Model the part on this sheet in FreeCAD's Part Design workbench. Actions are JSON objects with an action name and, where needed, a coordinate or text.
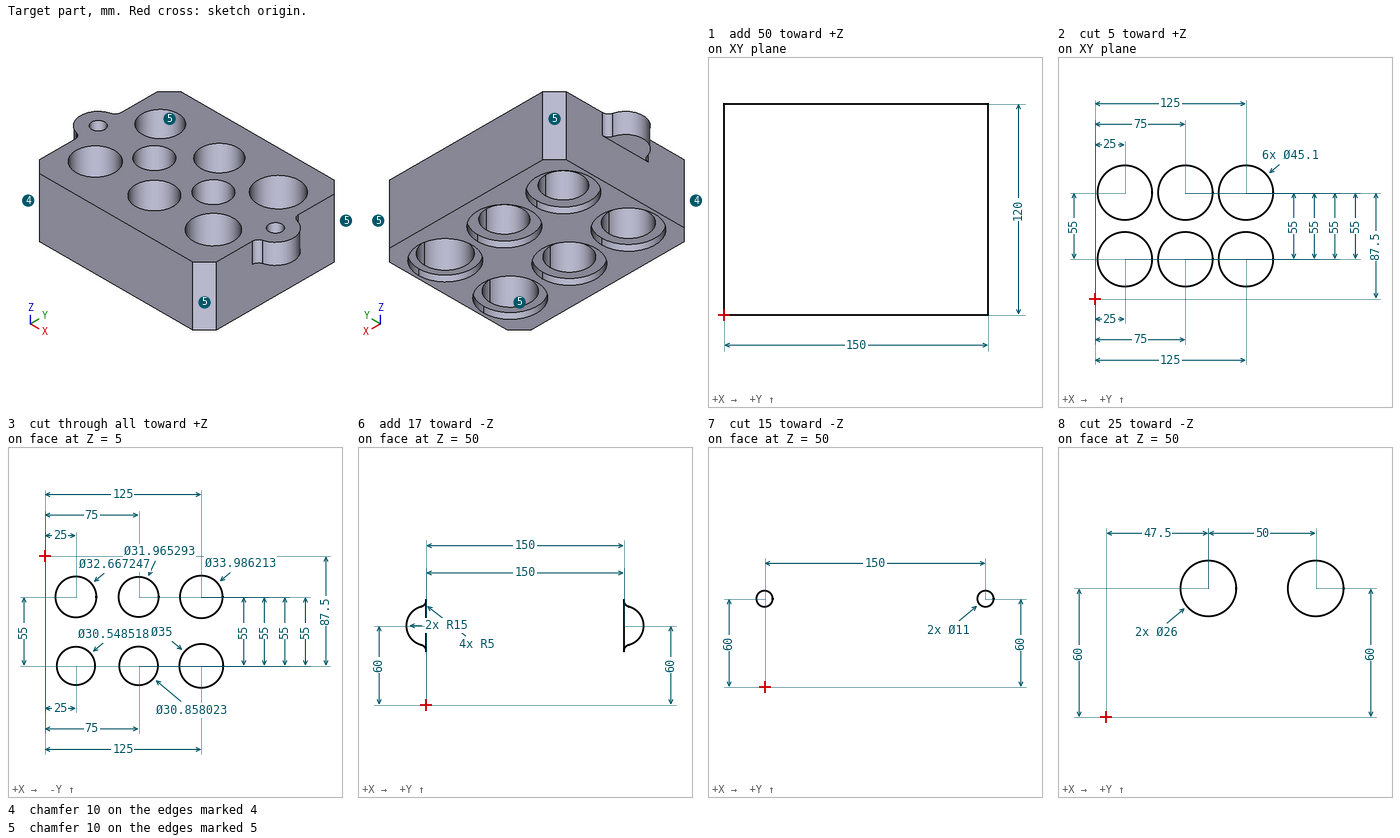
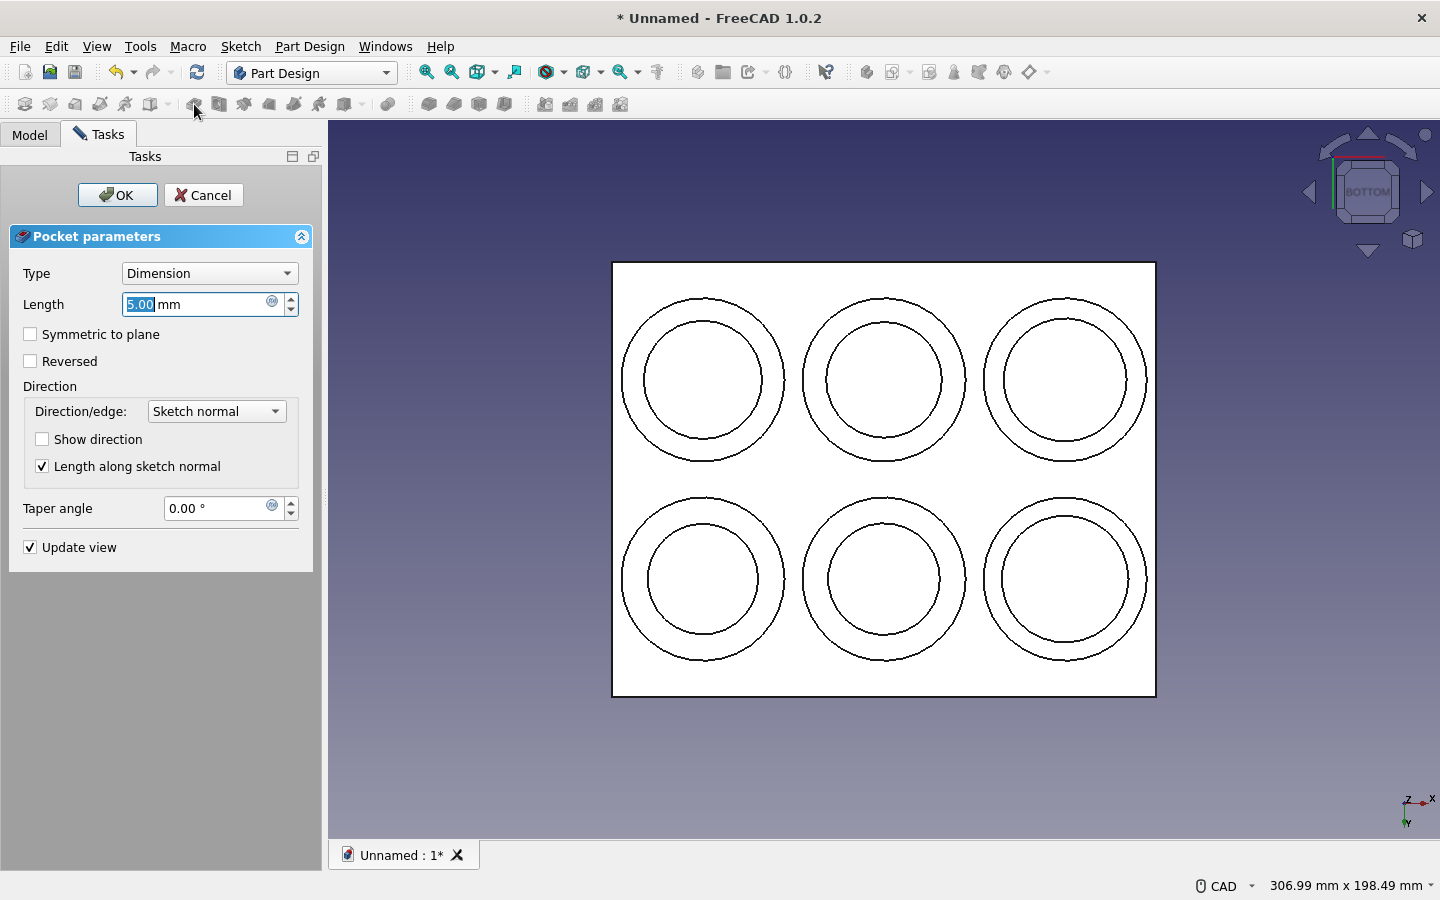
{"action": "left_click", "coordinate": [210, 274]}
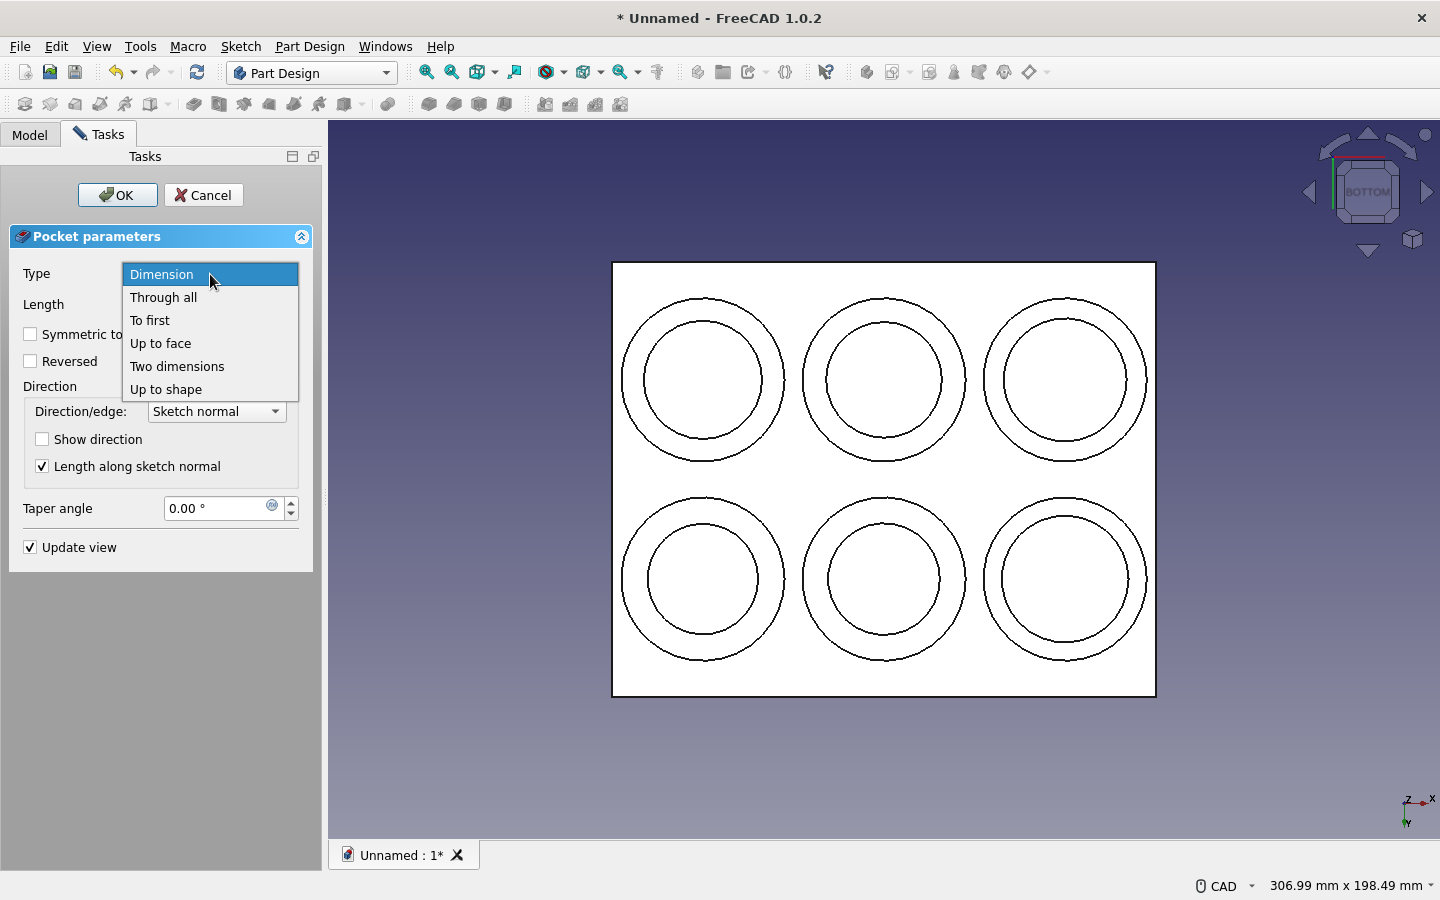
{"action": "left_click", "coordinate": [208, 298]}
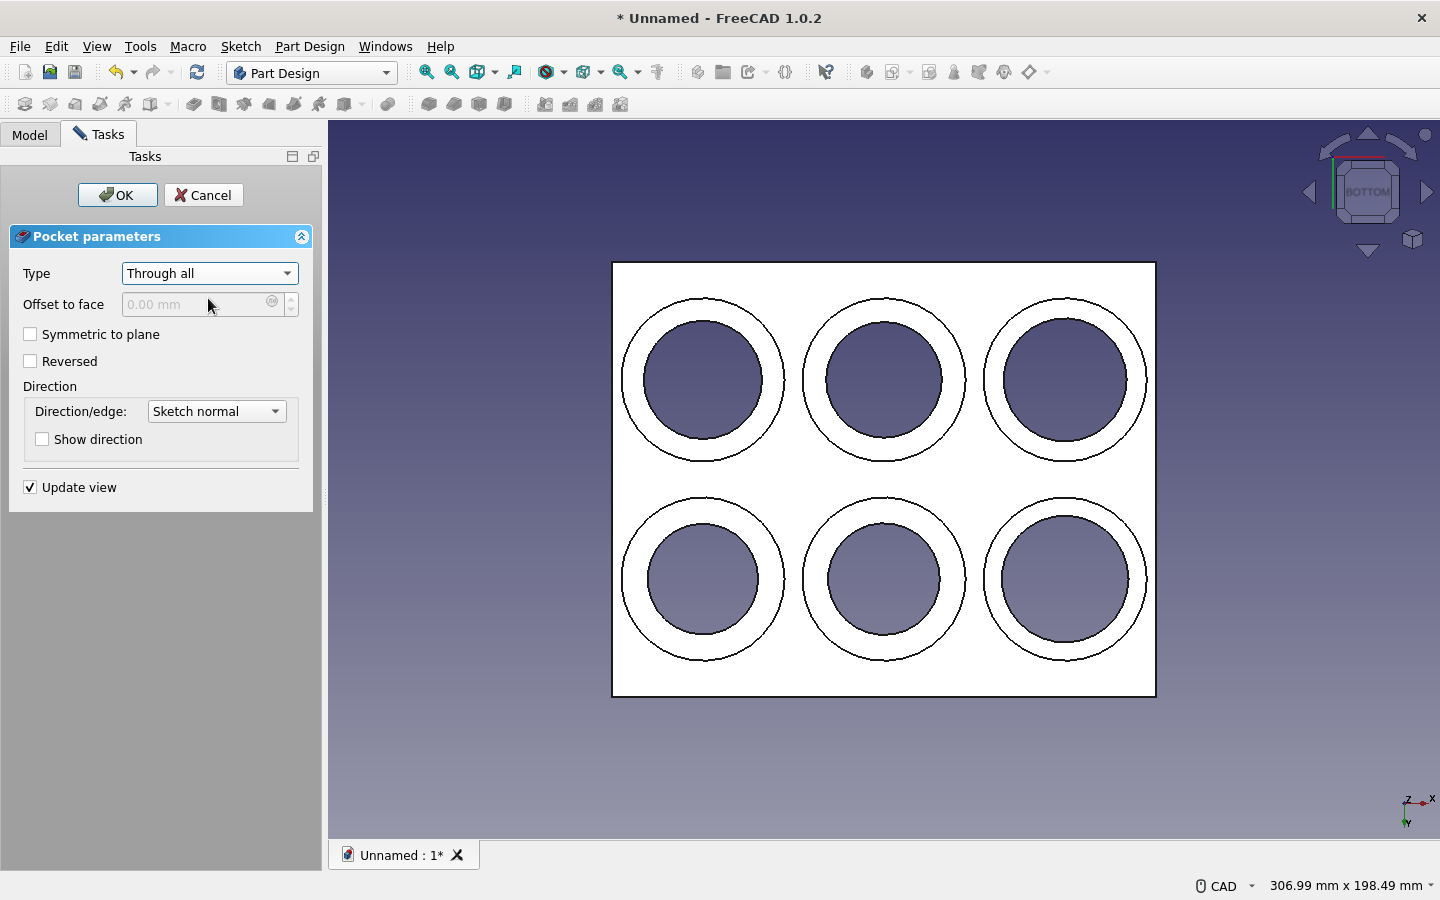
{"action": "left_click", "coordinate": [118, 195]}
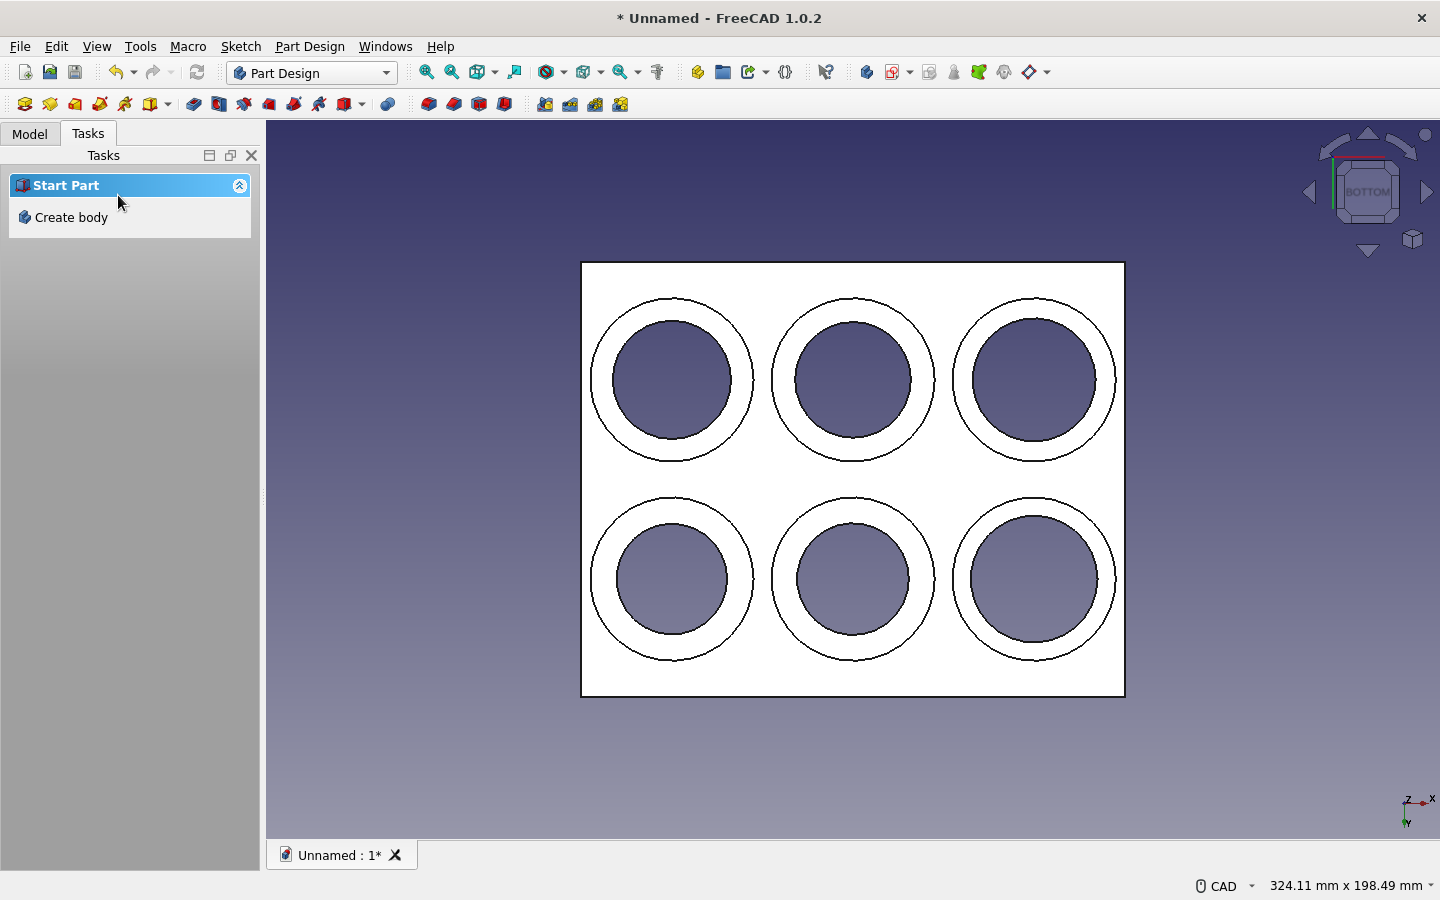
{"action": "key", "text": "0"}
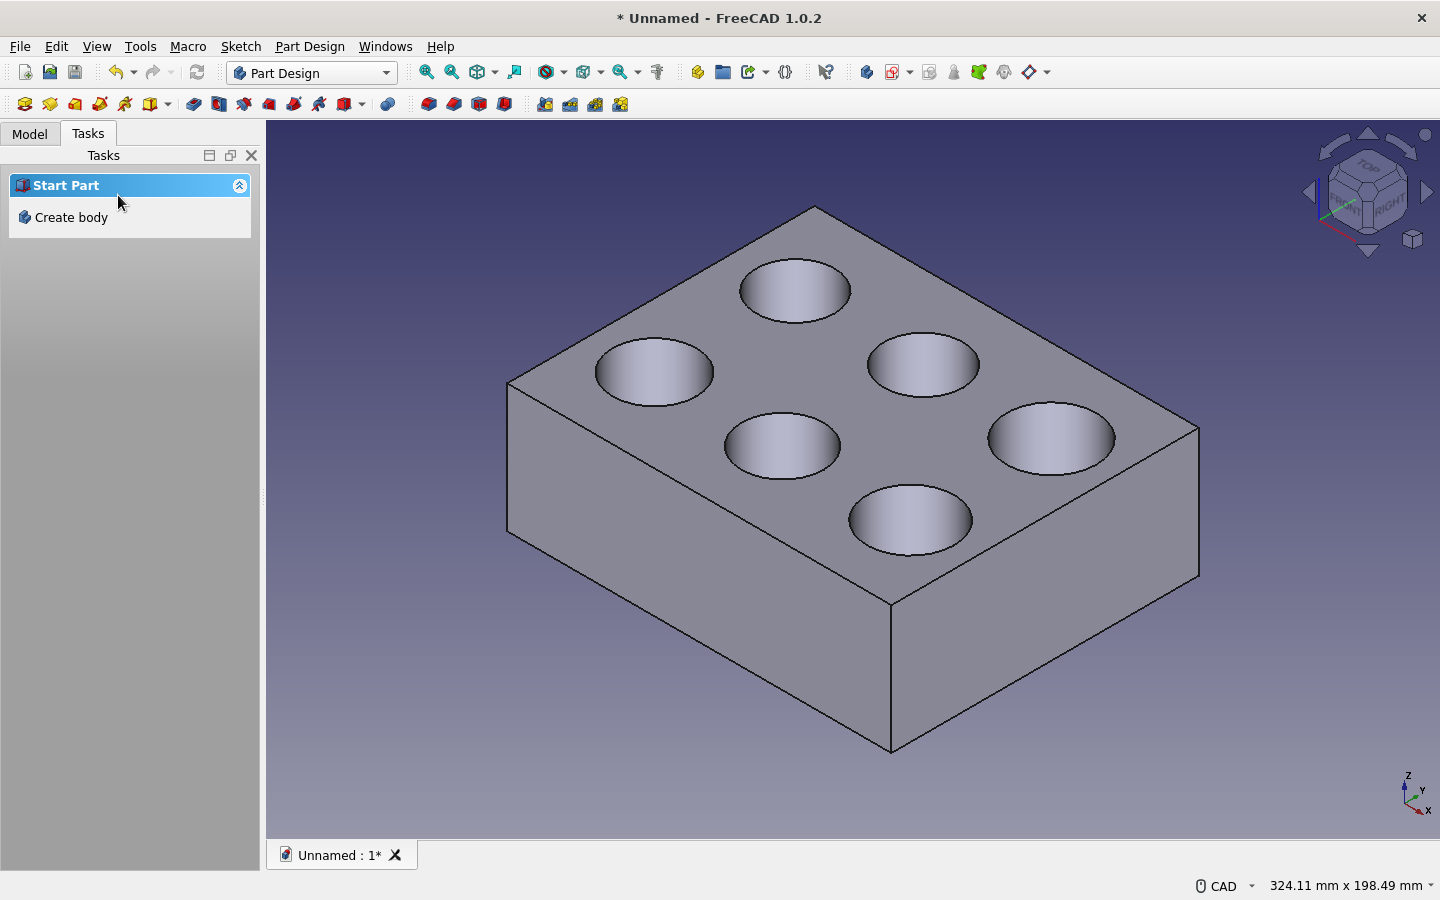
{"action": "key", "text": "2"}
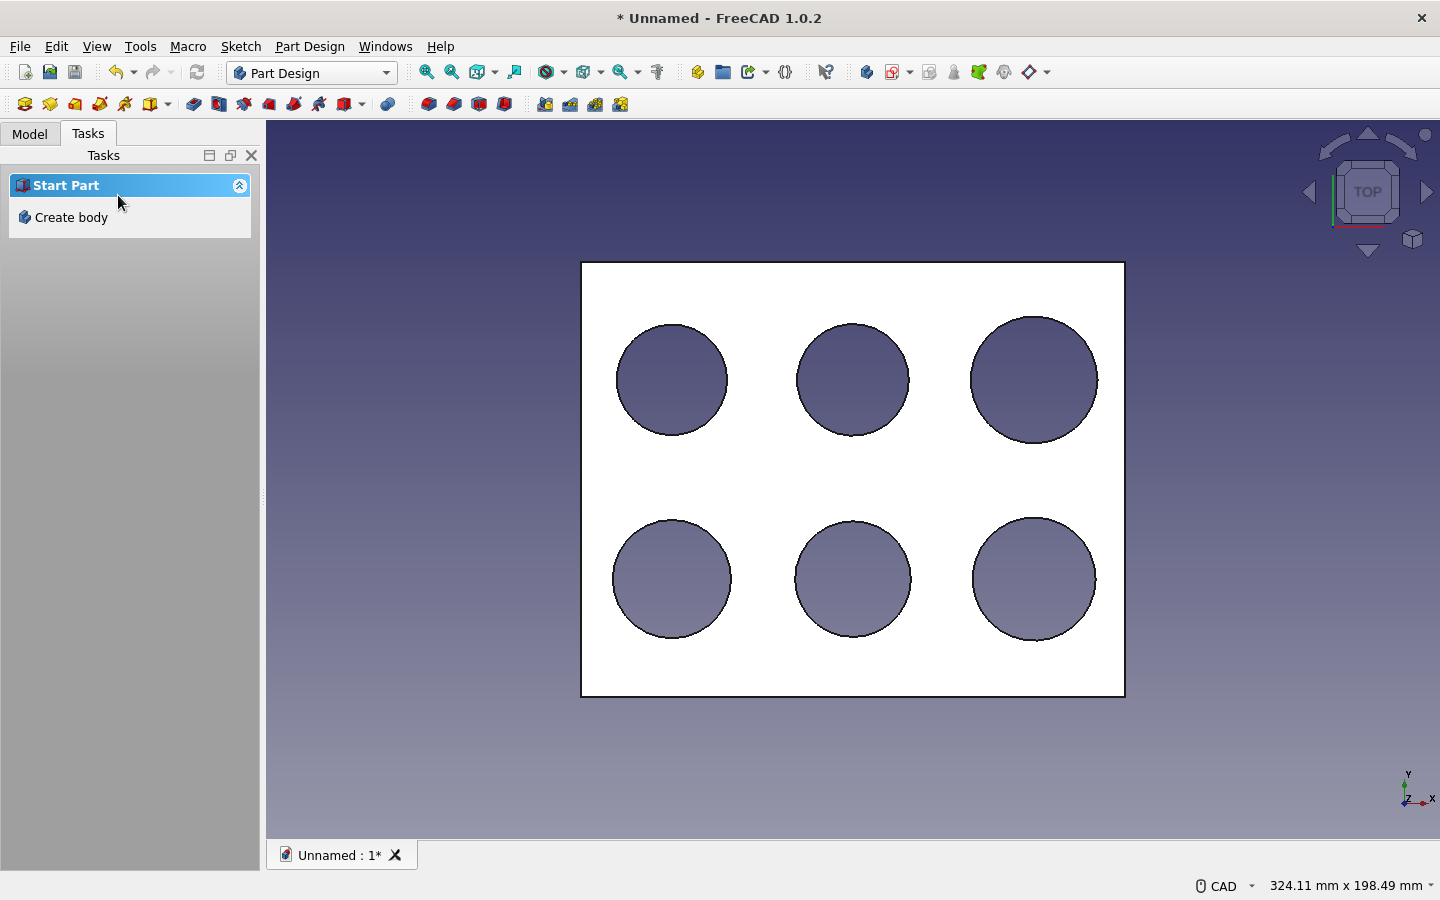
{"action": "key", "text": "1"}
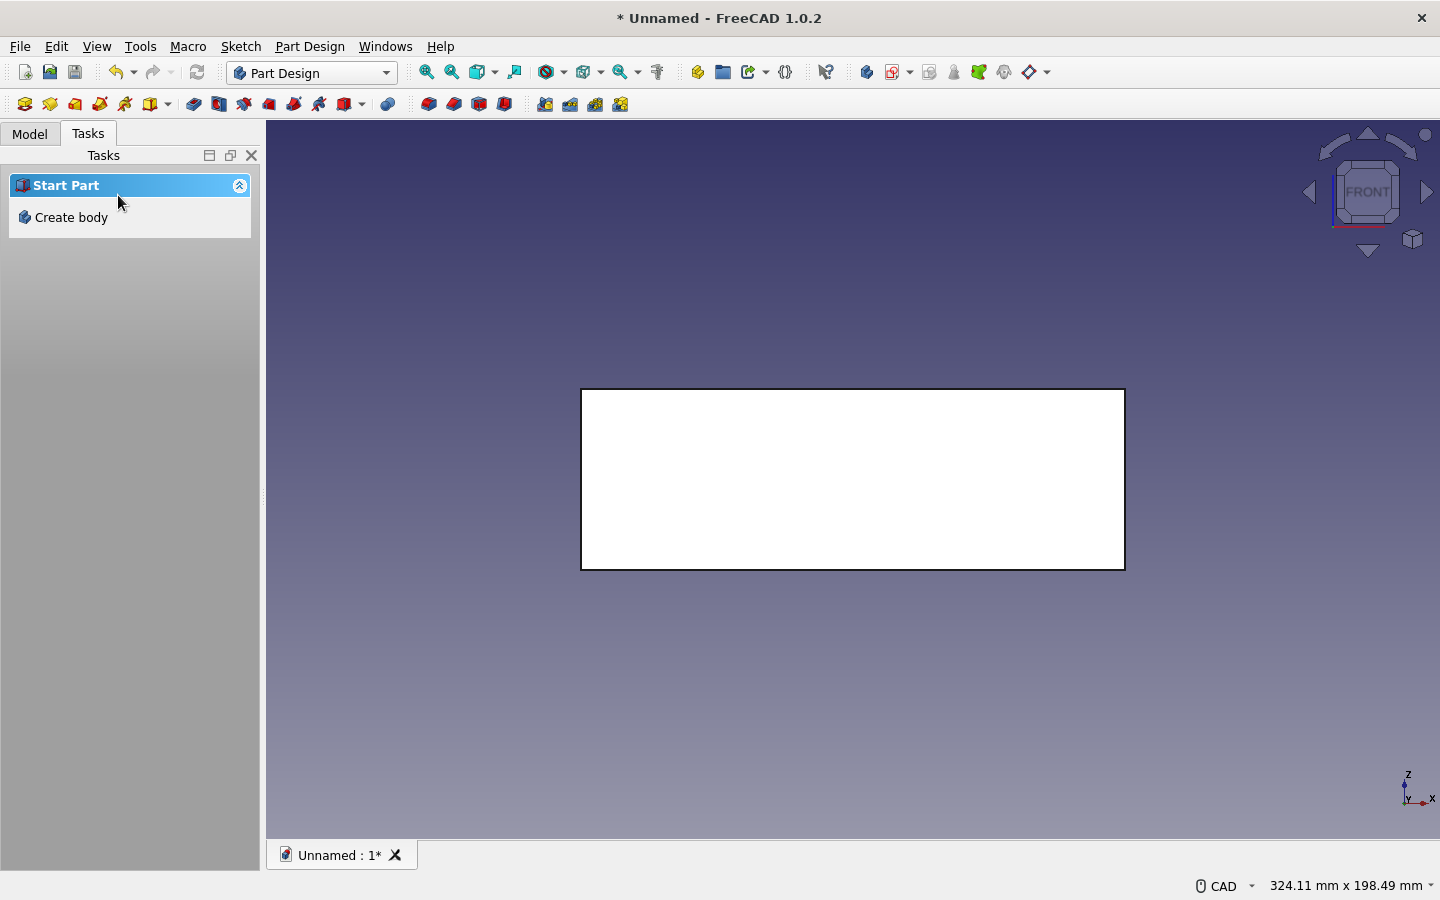
{"action": "left_click", "coordinate": [581, 478]}